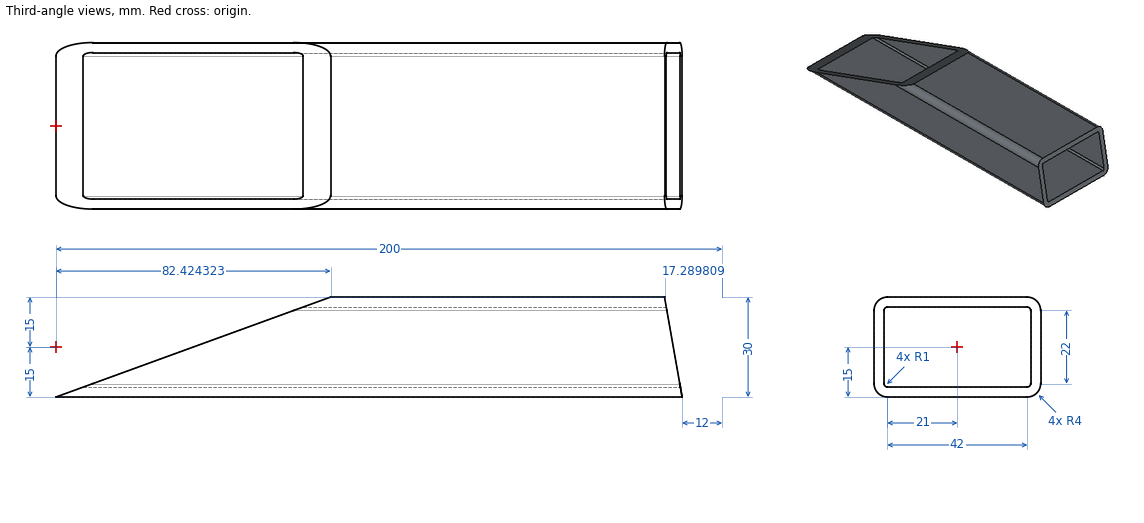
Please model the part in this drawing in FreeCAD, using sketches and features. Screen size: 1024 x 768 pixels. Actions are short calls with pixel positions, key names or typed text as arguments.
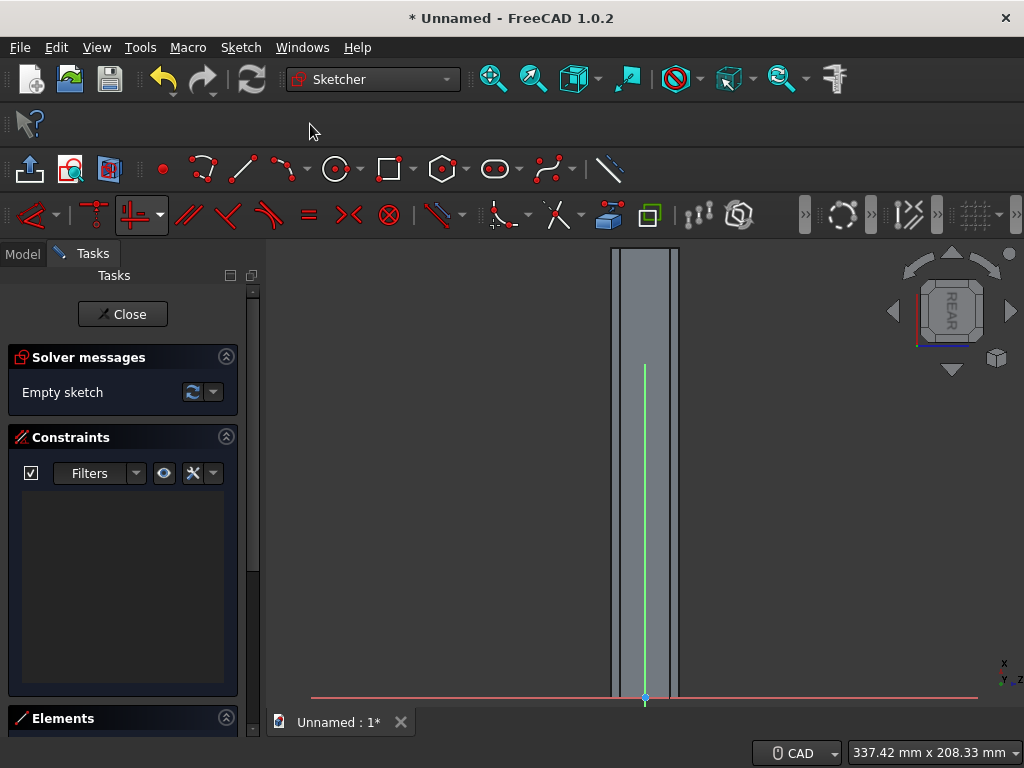
scroll(576, 473, down, 5)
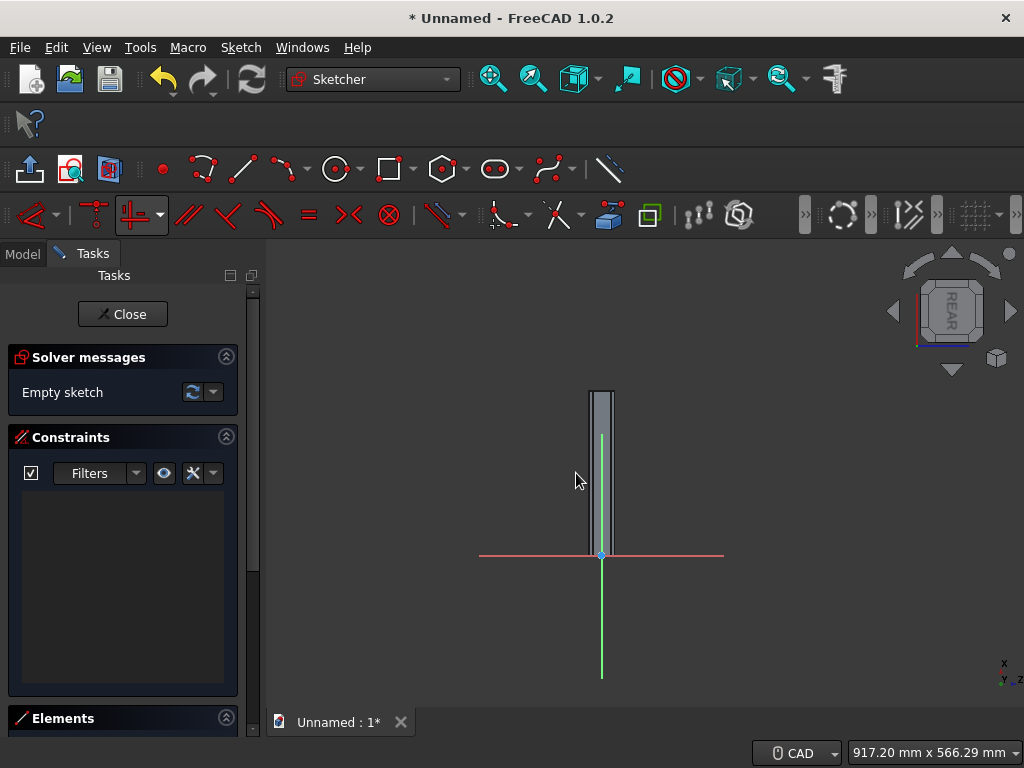
scroll(603, 393, up, 14)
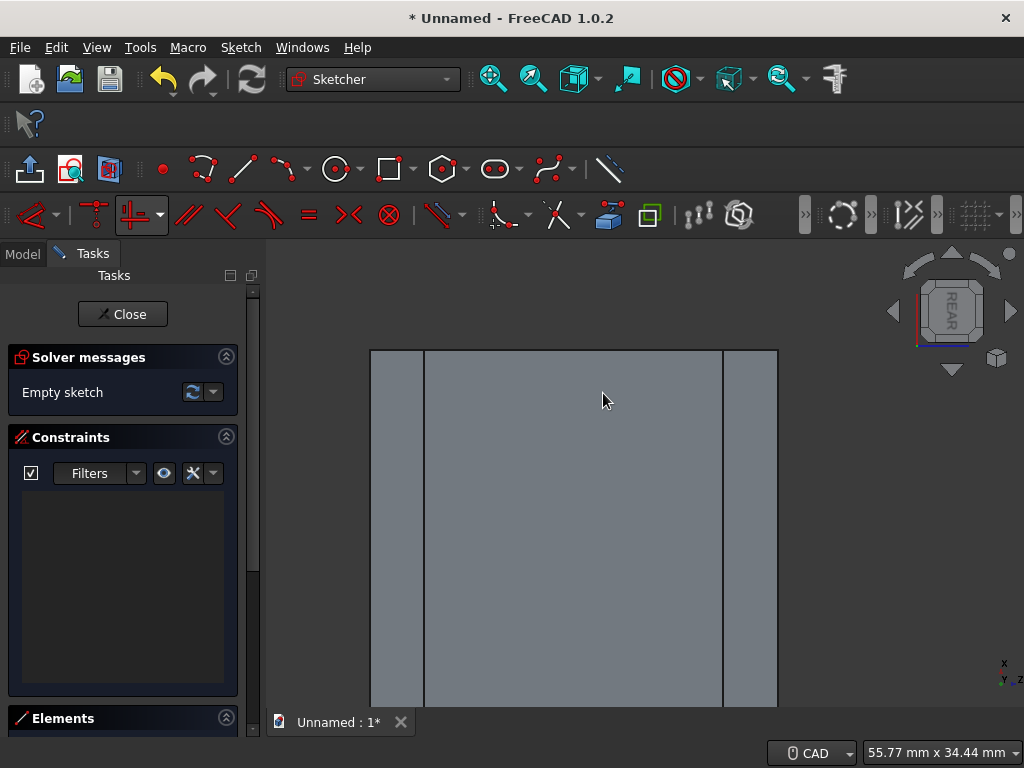
click(204, 170)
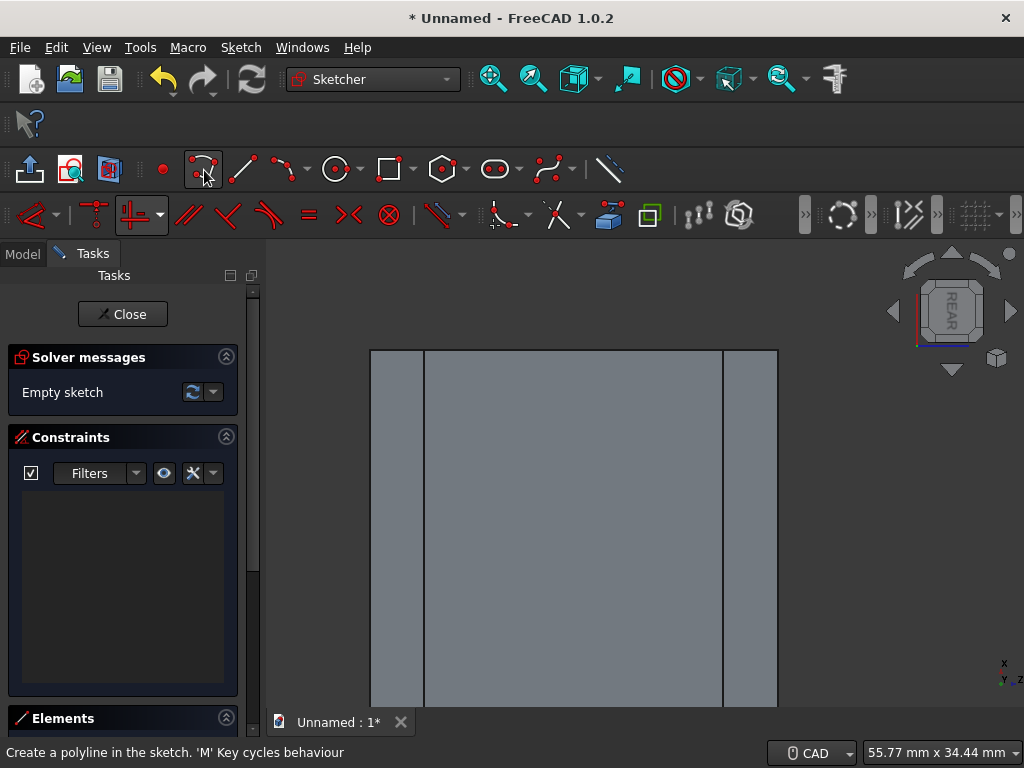
click(778, 585)
click(778, 350)
click(370, 350)
click(370, 513)
click(778, 586)
key(Escape)
key(Escape)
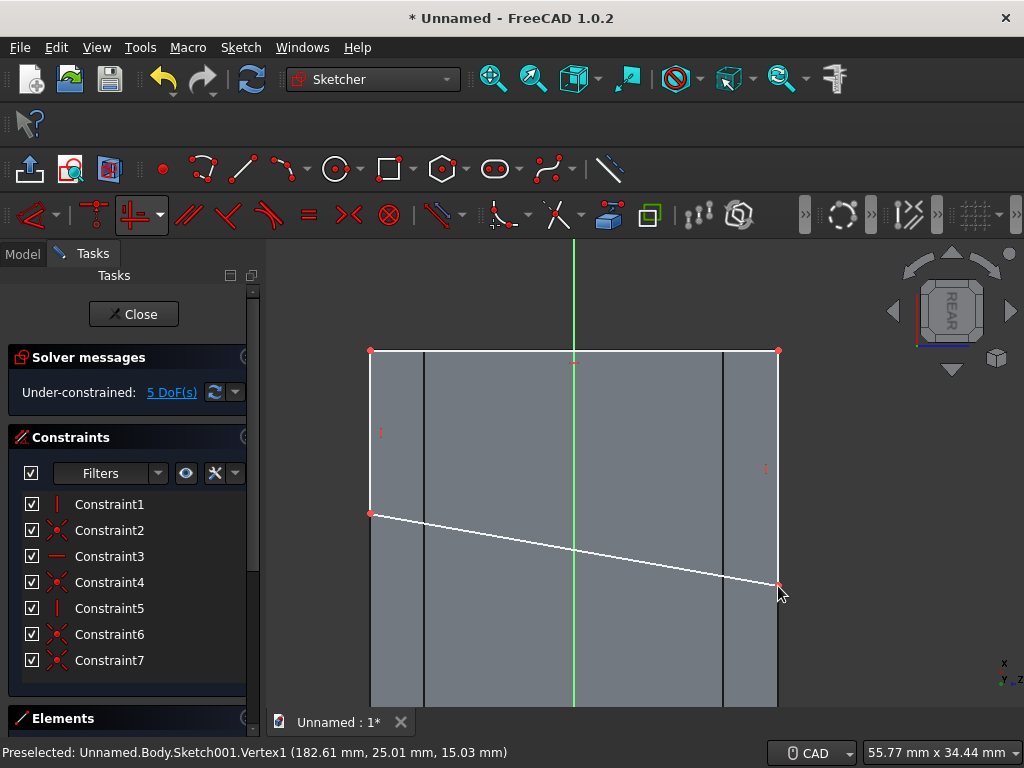
click(32, 216)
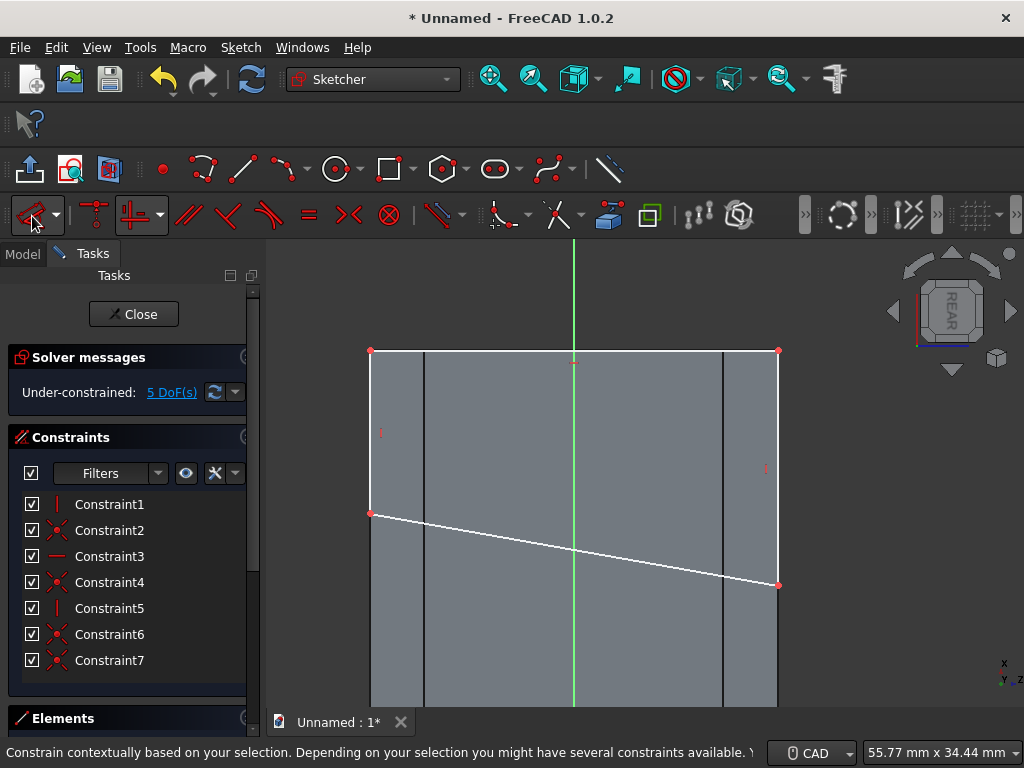
click(656, 351)
click(480, 317)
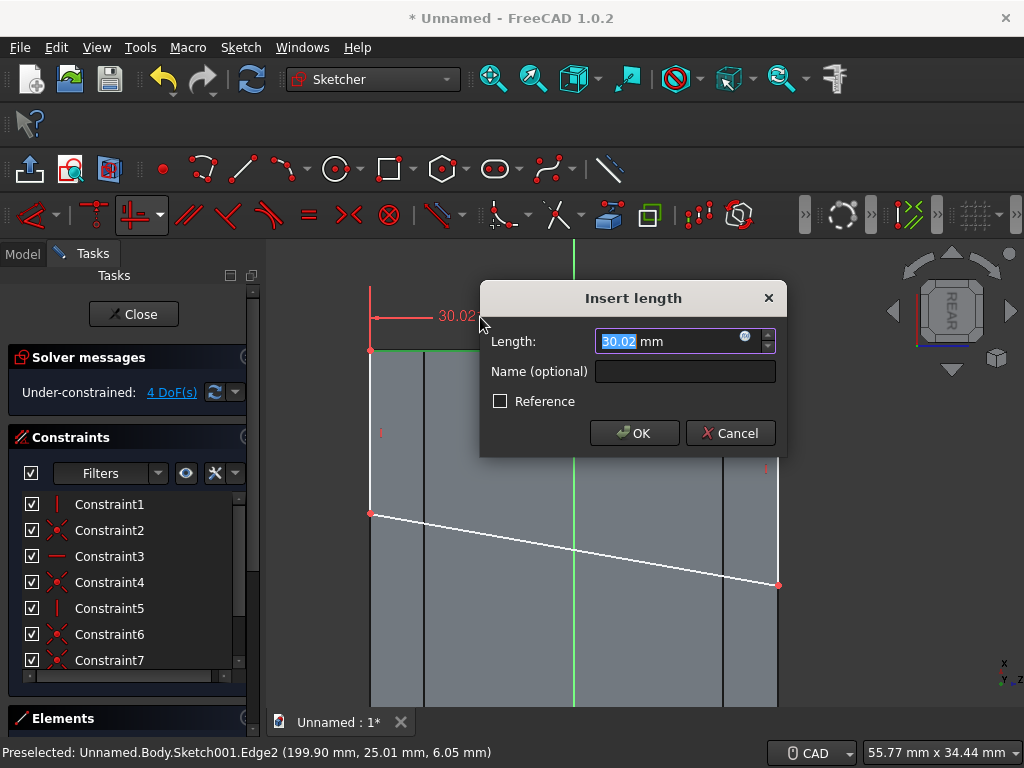
text(30)
key(Return)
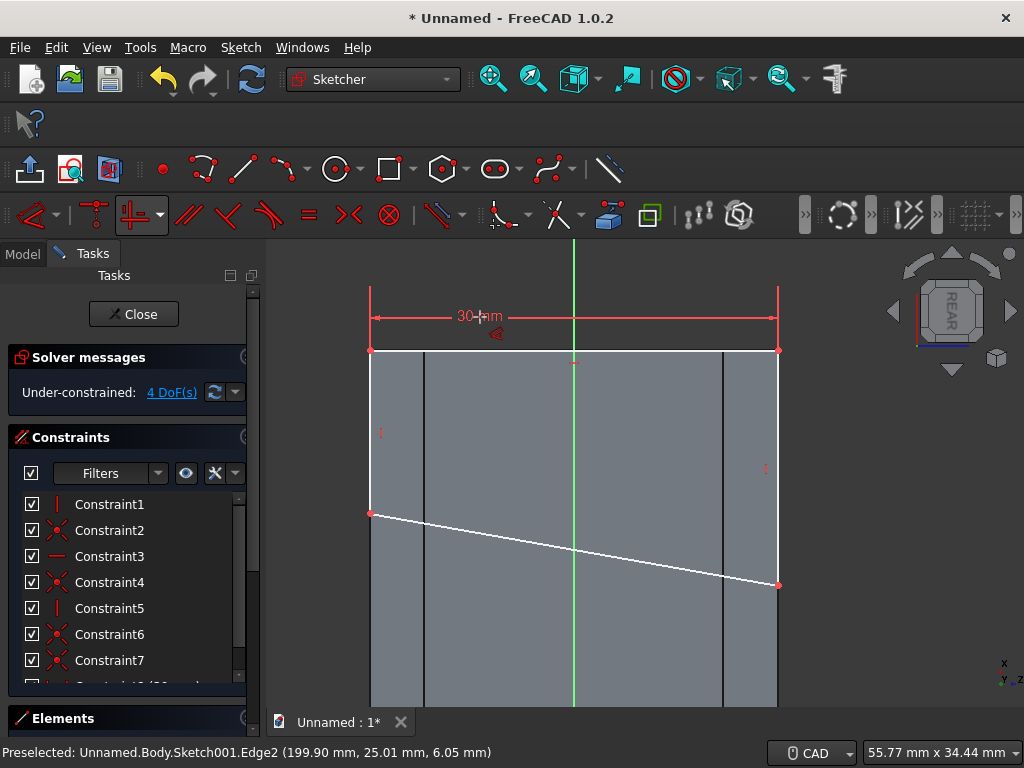
click(370, 400)
click(336, 432)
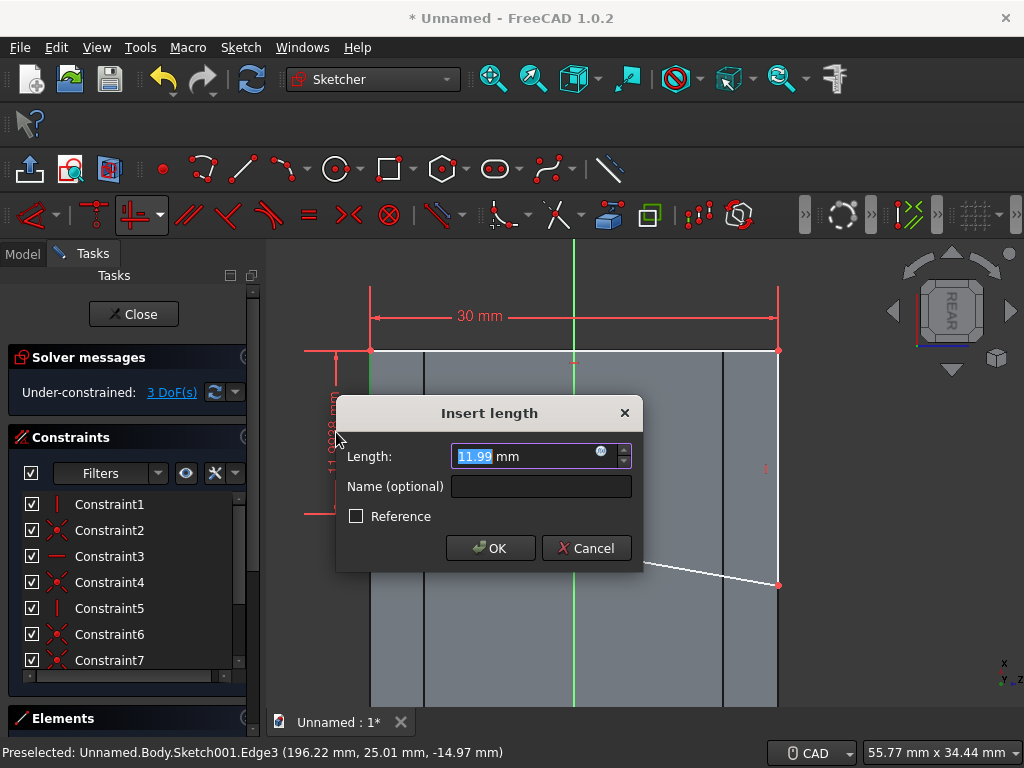
text(12)
key(Return)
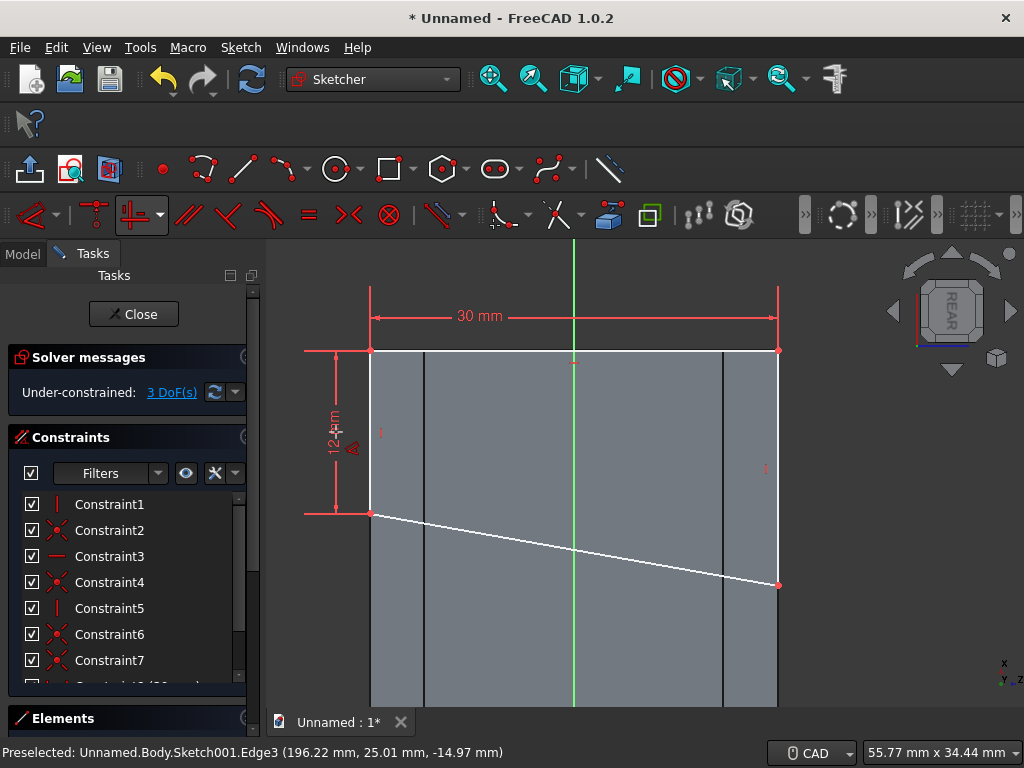
click(778, 586)
click(676, 552)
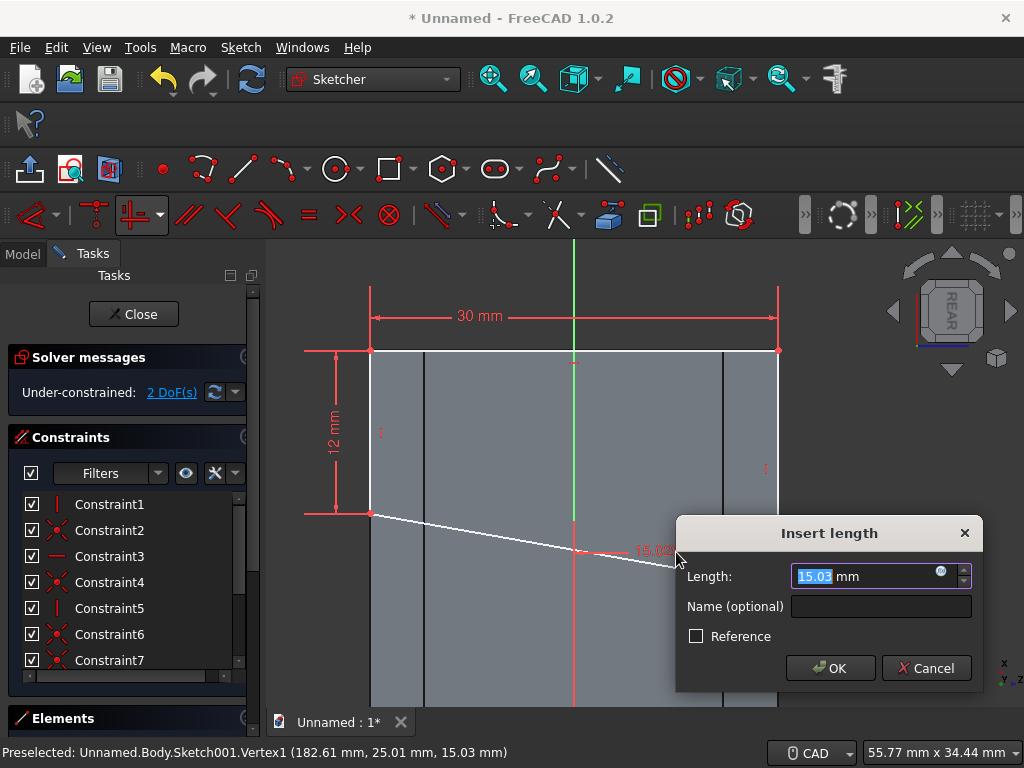
text(15)
key(Return)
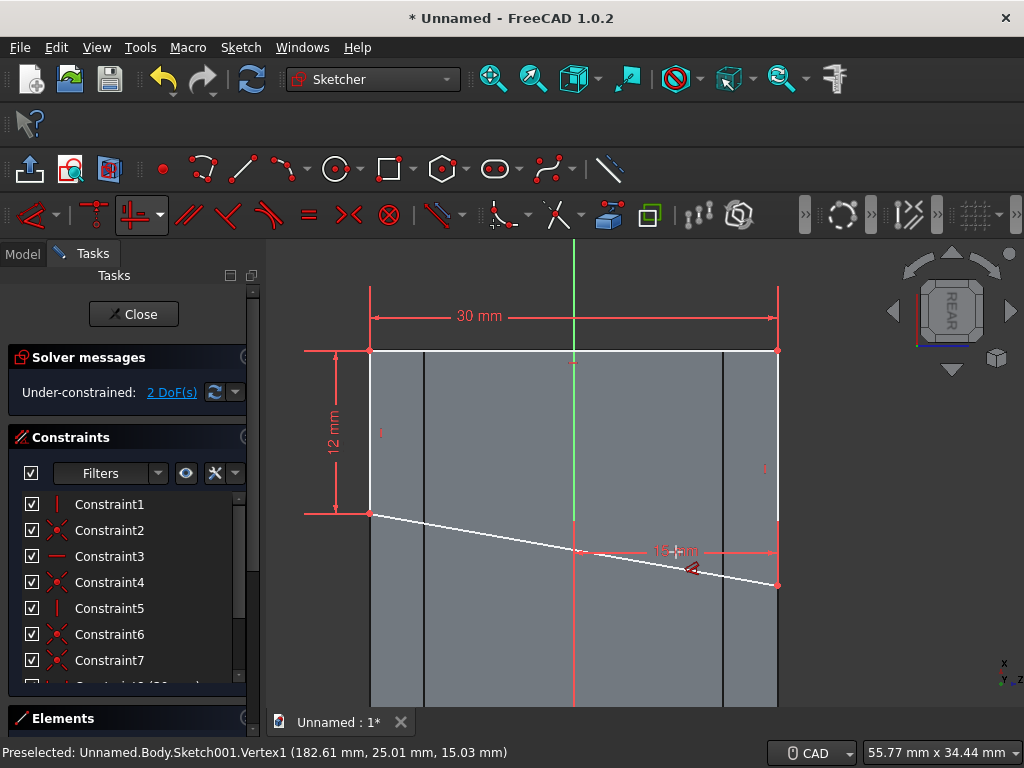
click(778, 351)
click(812, 515)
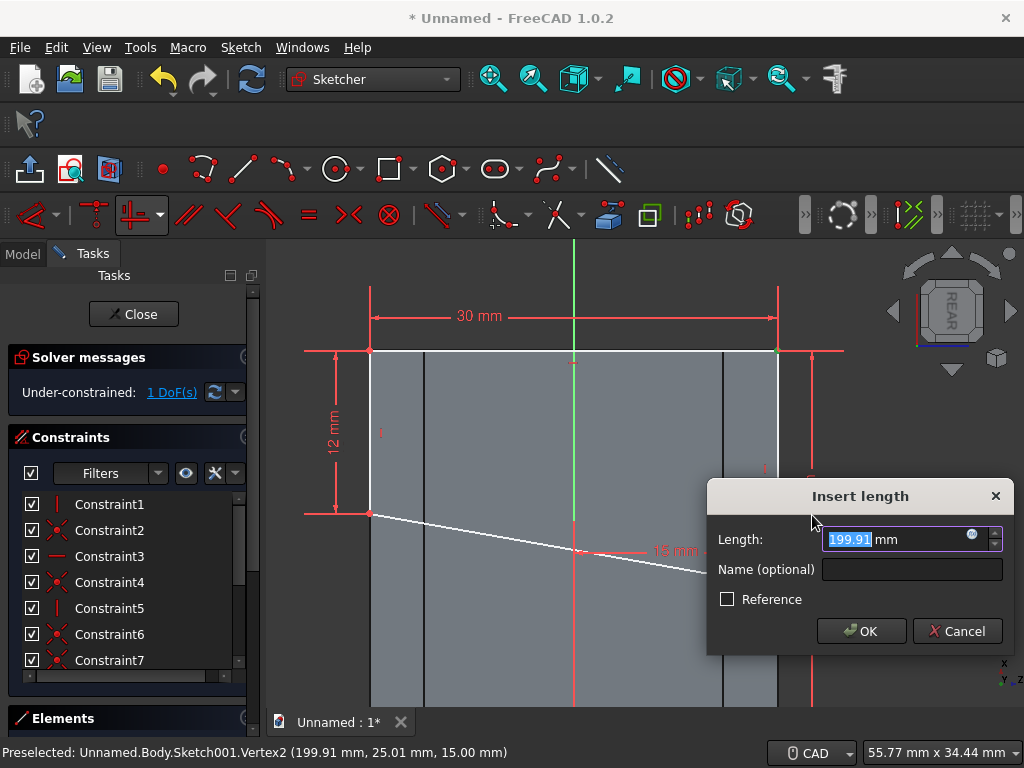
text(200)
key(Return)